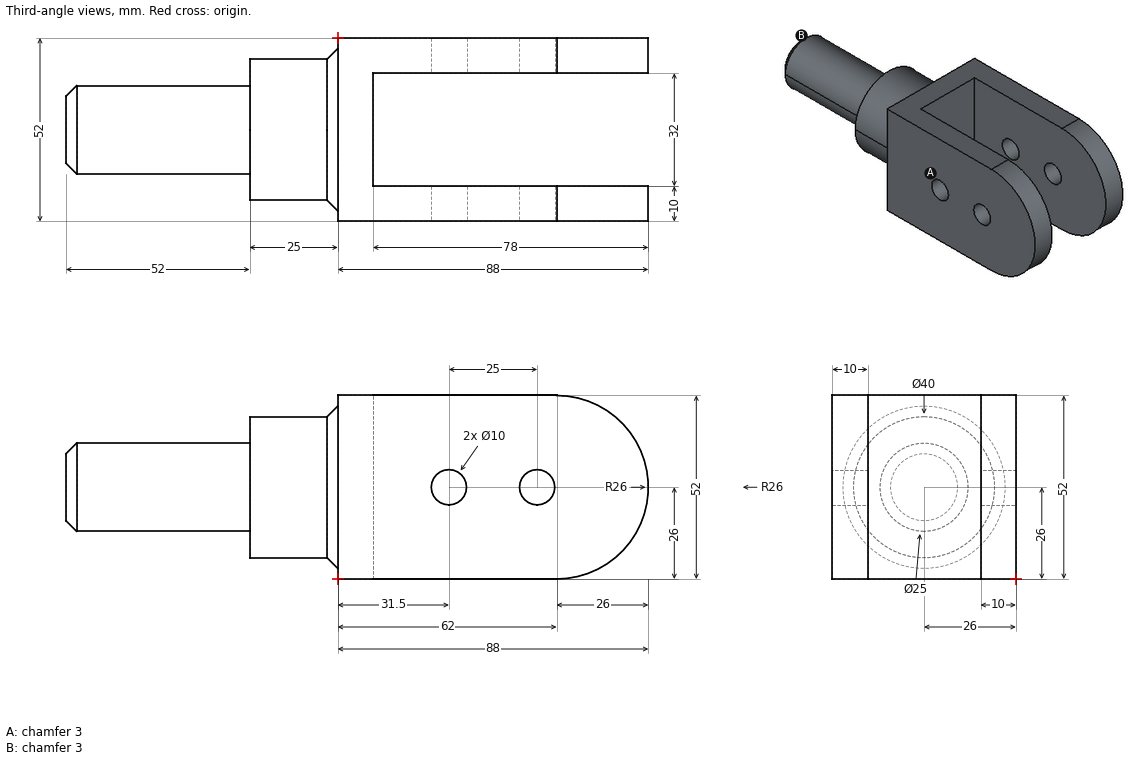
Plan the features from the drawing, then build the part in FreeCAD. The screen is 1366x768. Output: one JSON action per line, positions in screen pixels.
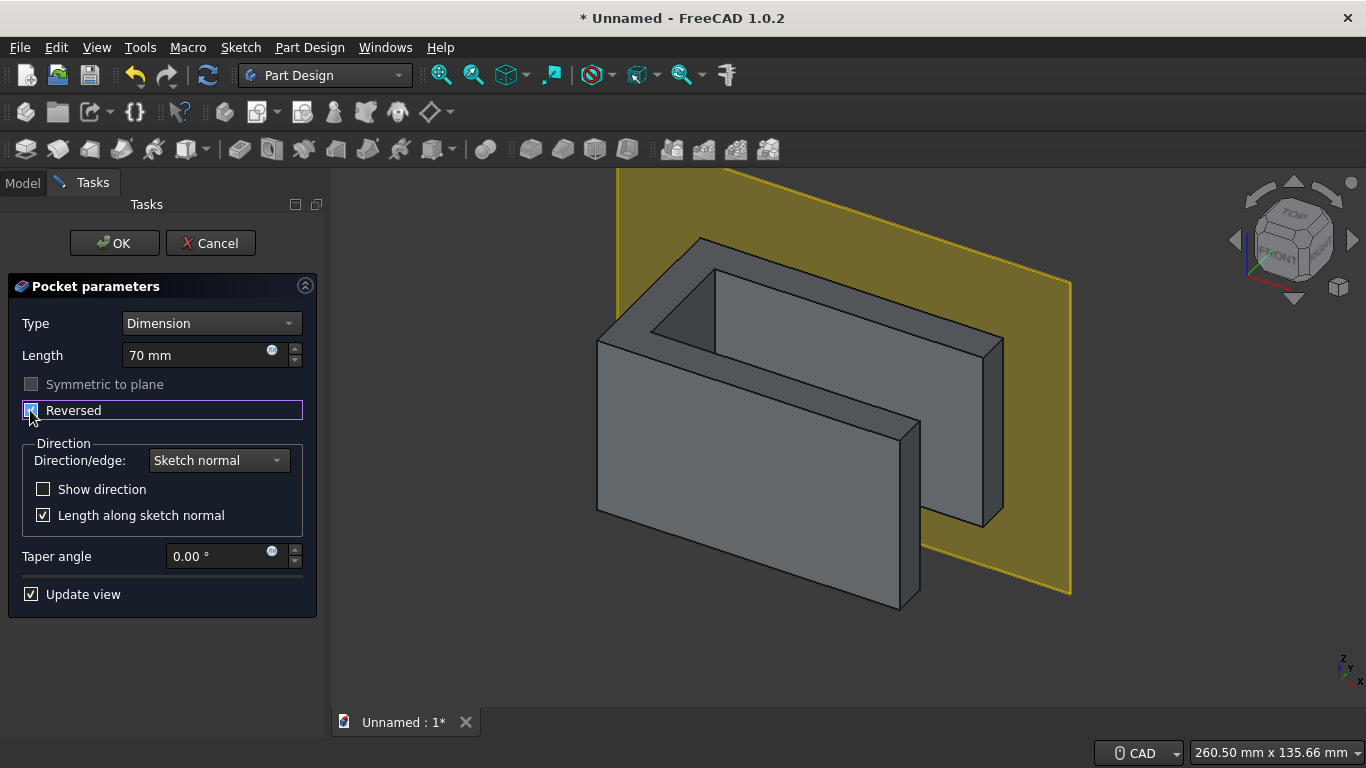
{"action": "left_click", "coordinate": [115, 243]}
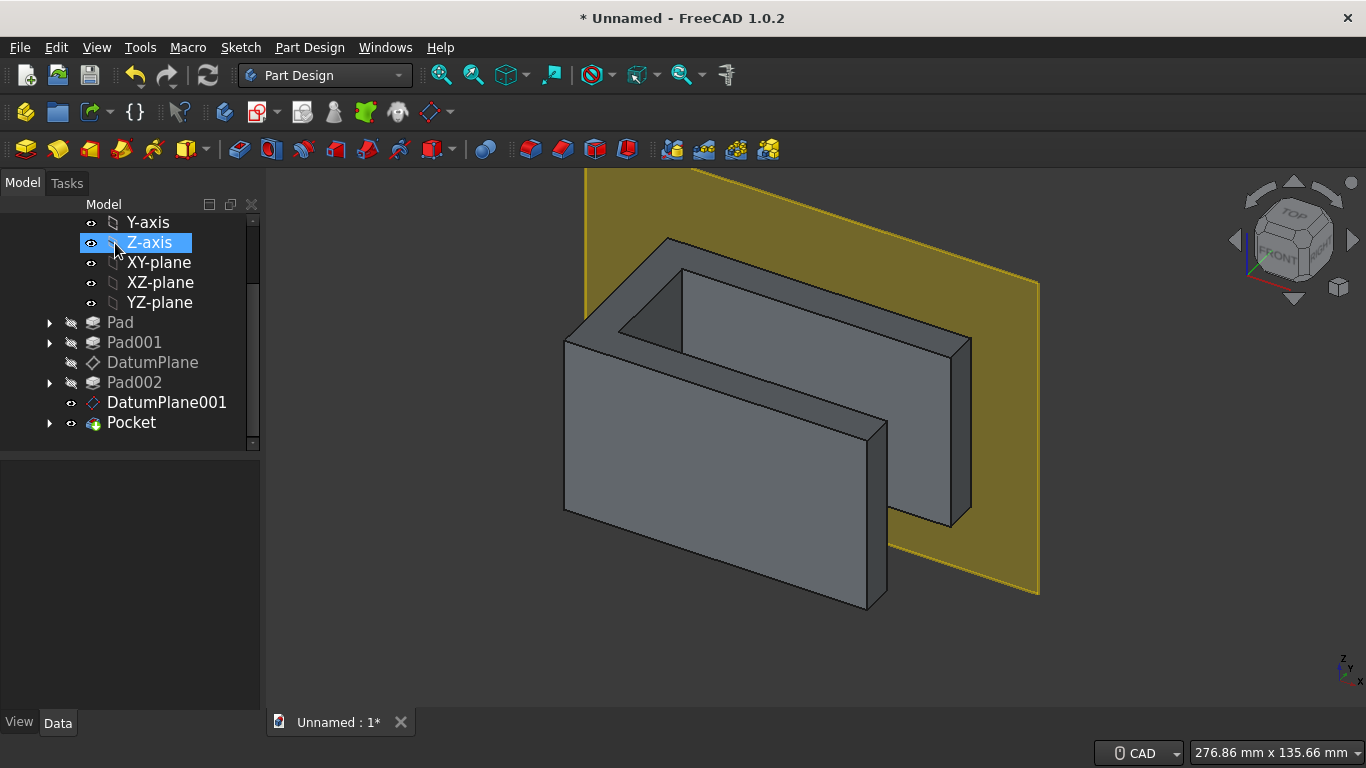
{"action": "left_click", "coordinate": [116, 403]}
{"action": "key", "text": "space"}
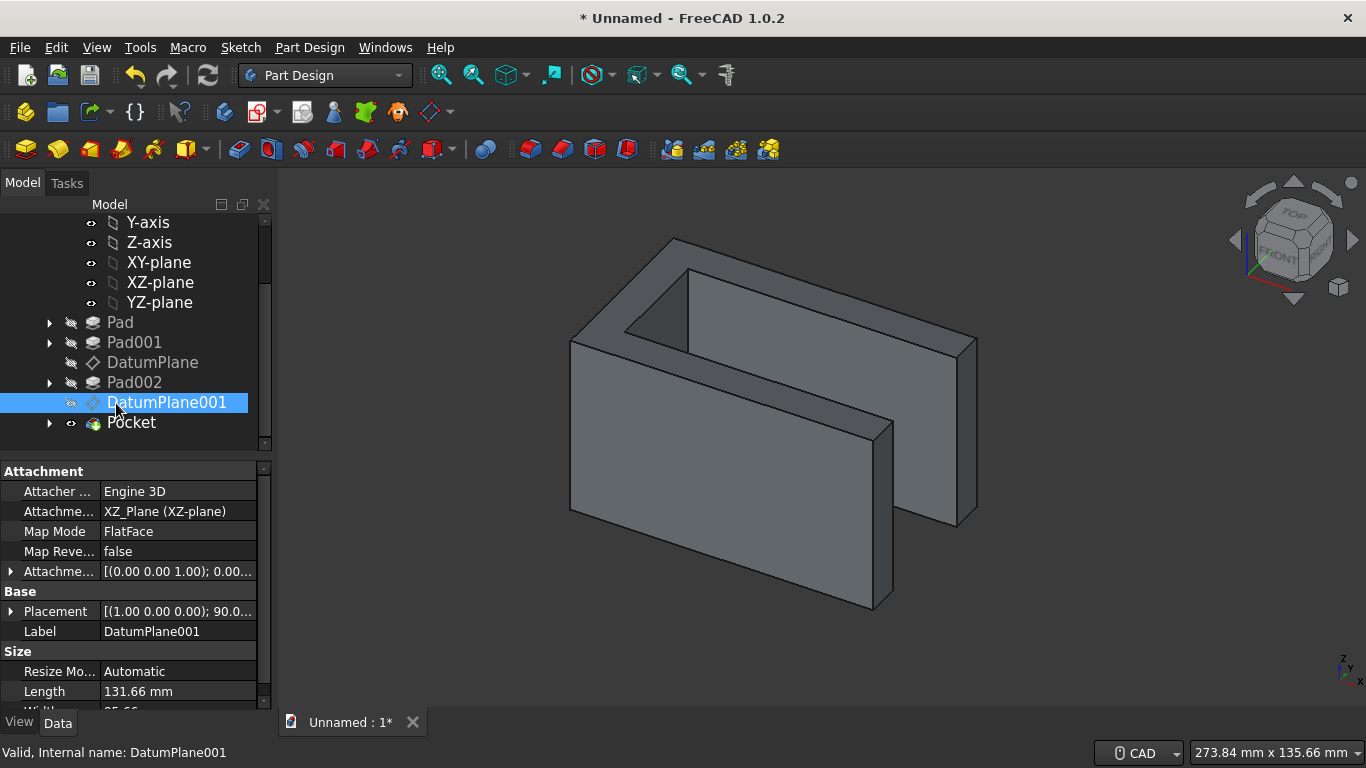
{"action": "left_click", "coordinate": [765, 489]}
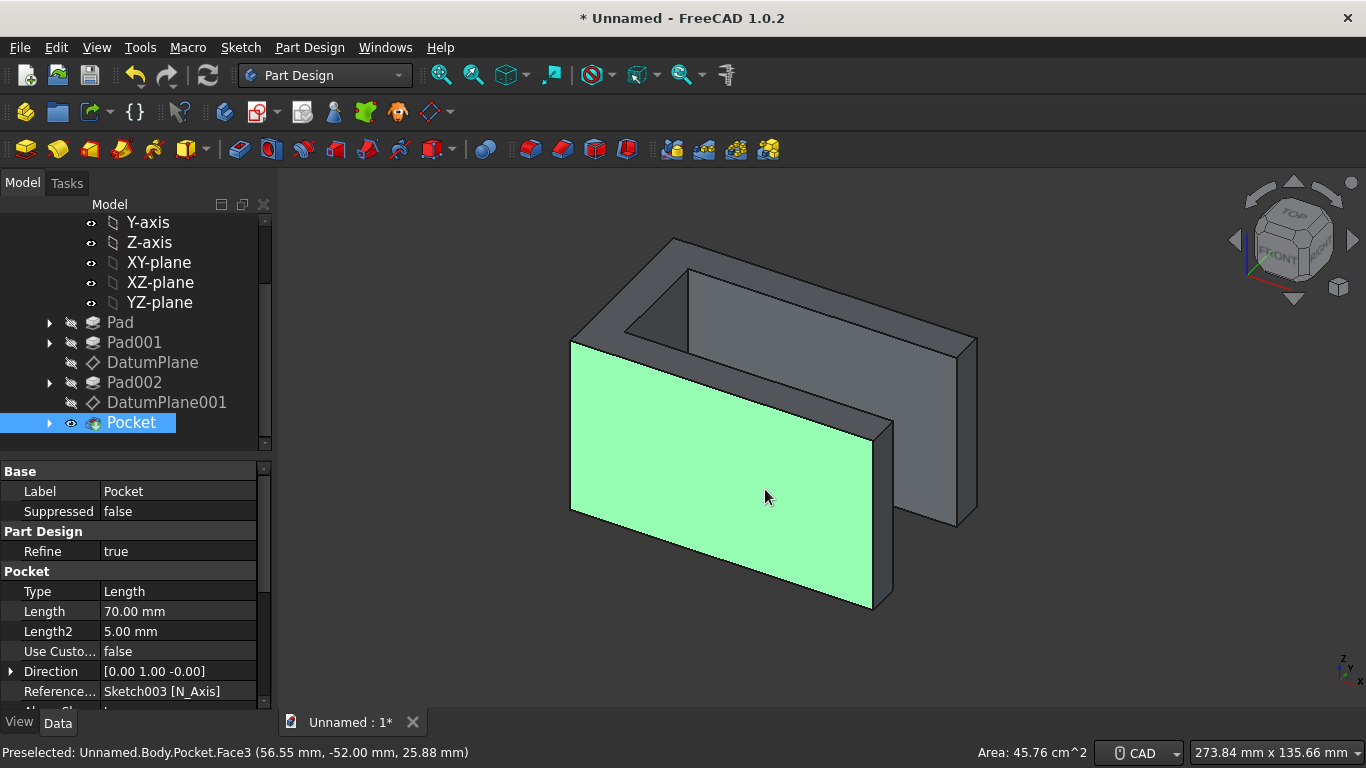
{"action": "left_click", "coordinate": [258, 112]}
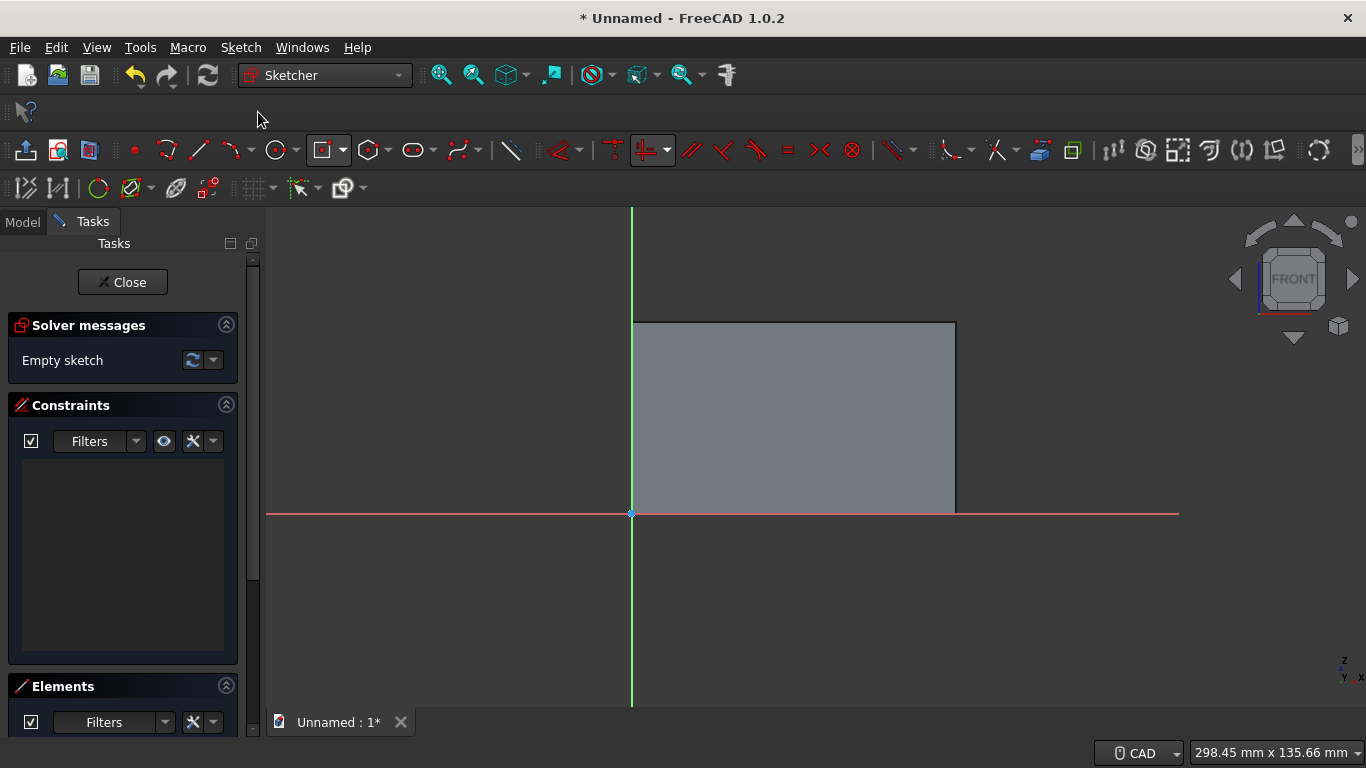
{"action": "scroll", "coordinate": [889, 338], "scroll_direction": "up", "scroll_amount": 2}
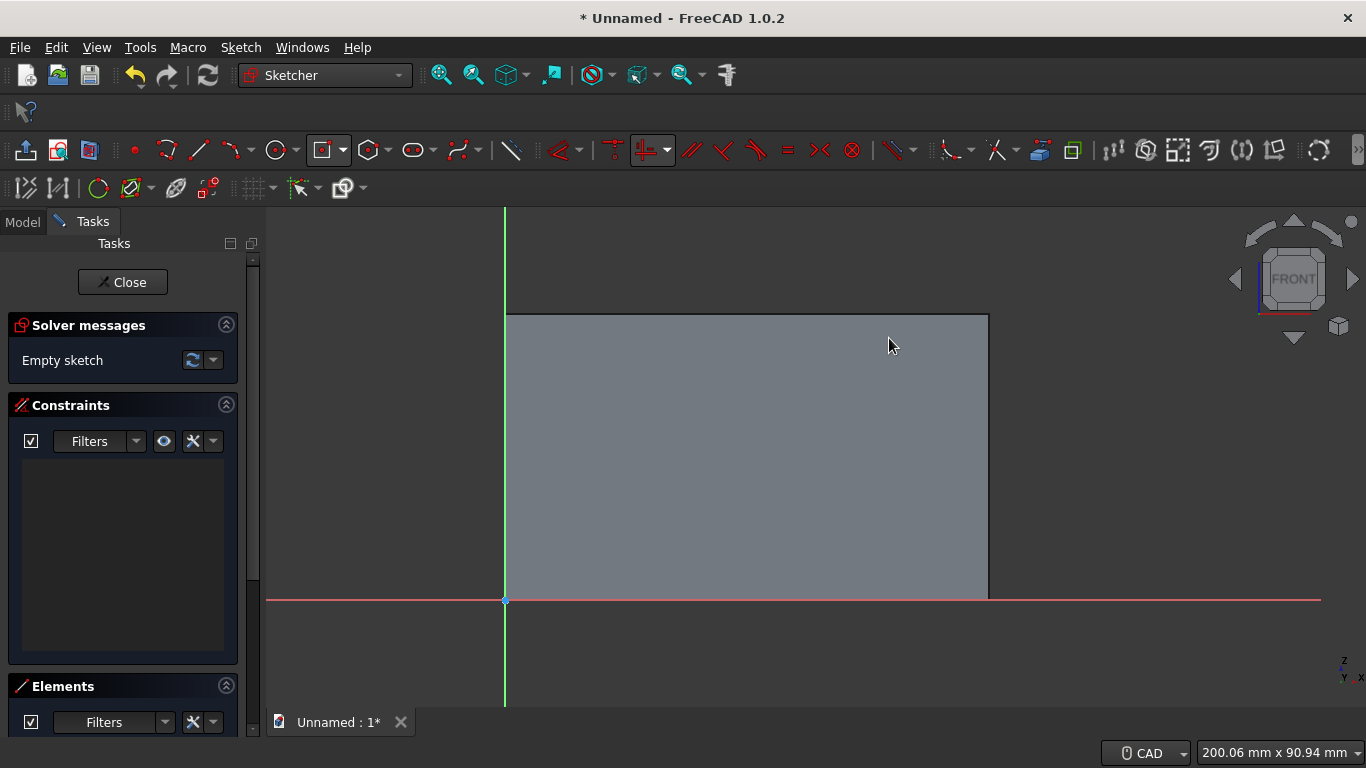
{"action": "key", "text": "g r"}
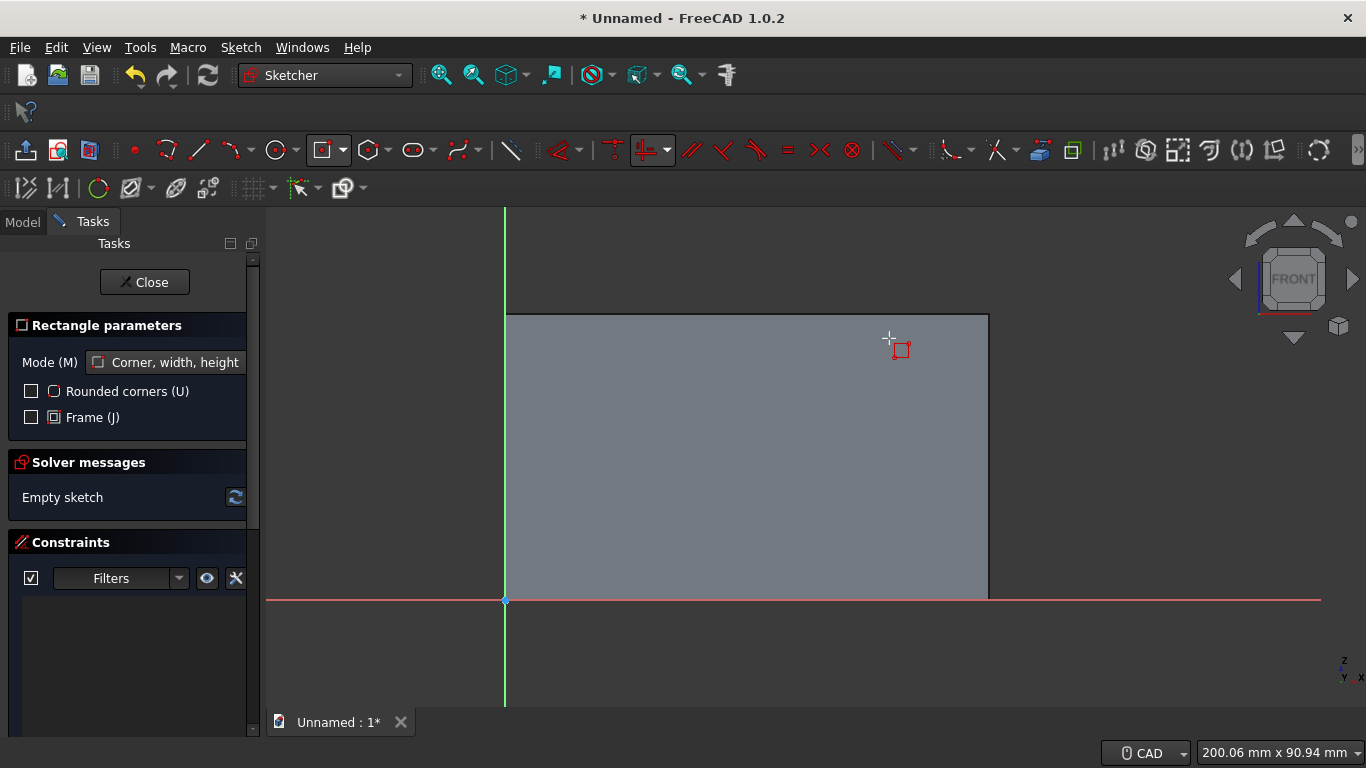
{"action": "left_click", "coordinate": [846, 314]}
{"action": "left_click", "coordinate": [989, 600]}
{"action": "key", "text": "Escape"}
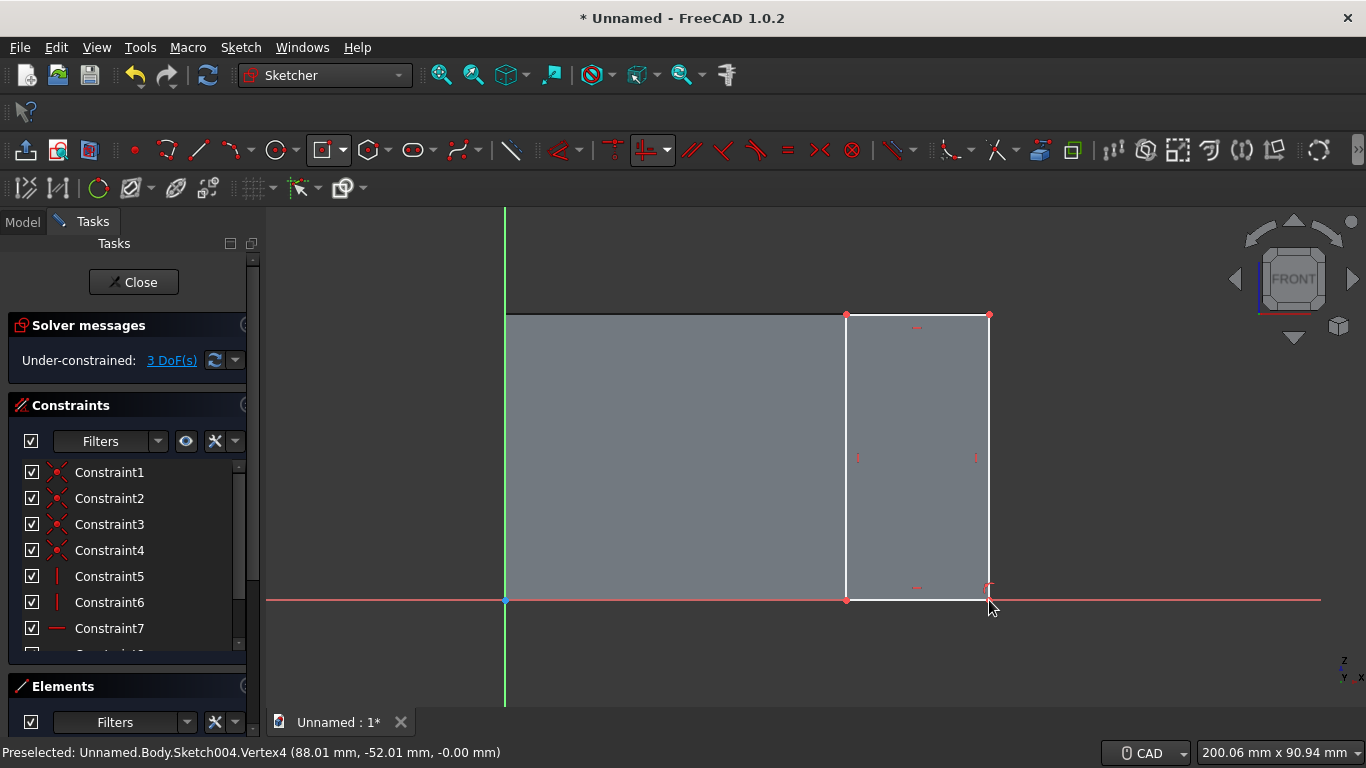
{"action": "left_click", "coordinate": [558, 150]}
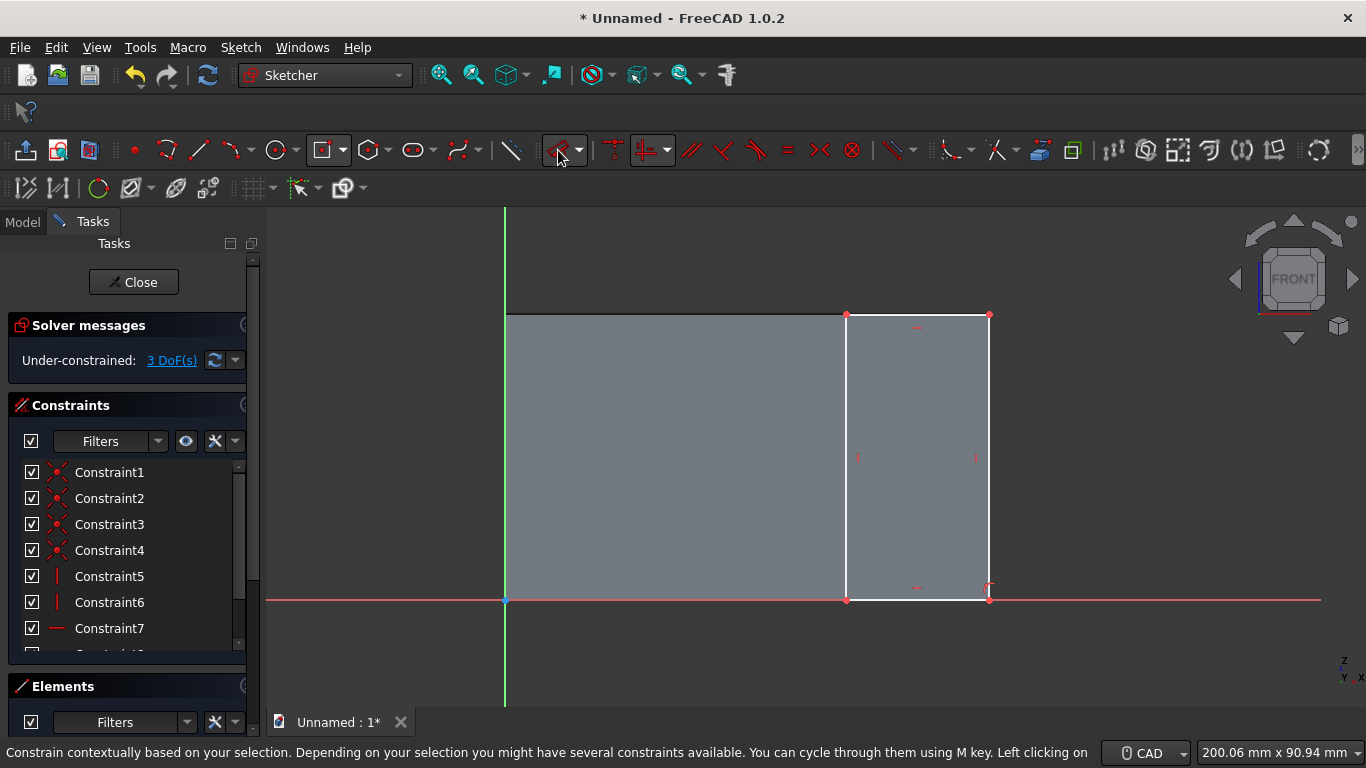
{"action": "left_click", "coordinate": [846, 401]}
{"action": "left_click", "coordinate": [880, 458]}